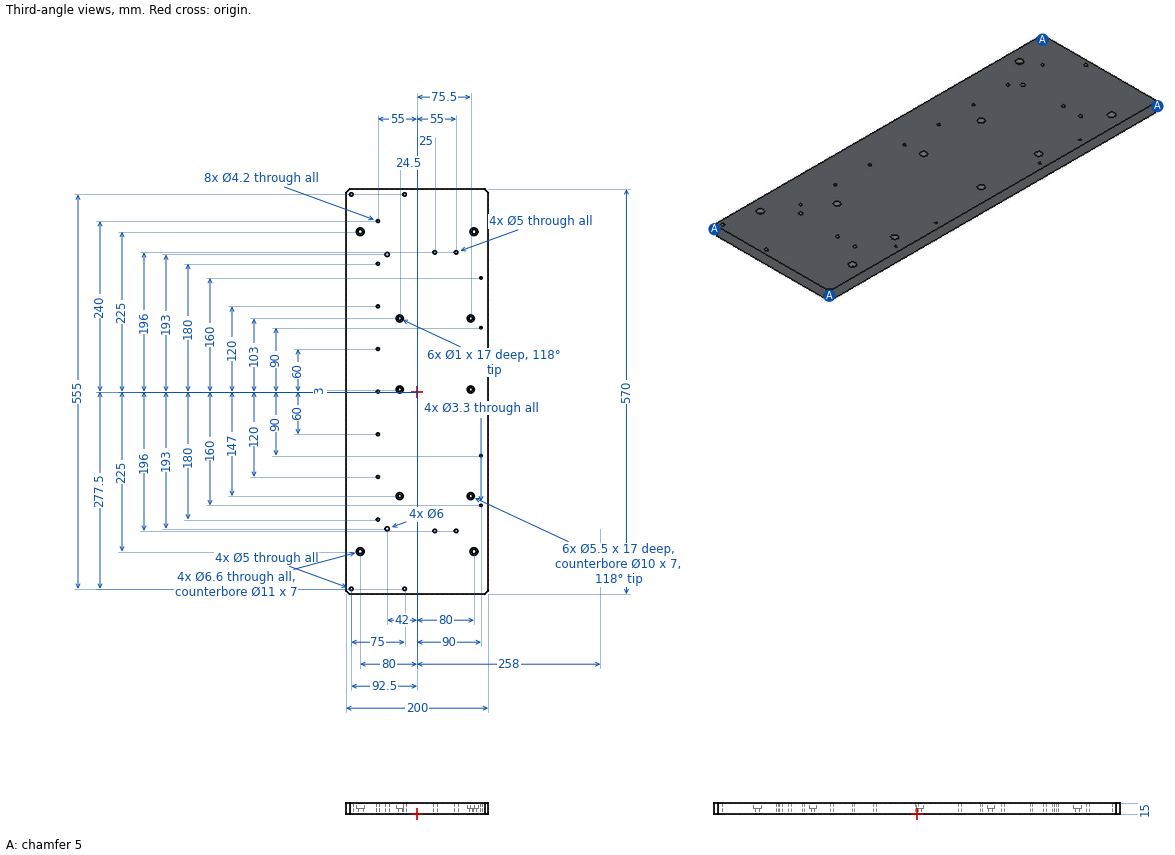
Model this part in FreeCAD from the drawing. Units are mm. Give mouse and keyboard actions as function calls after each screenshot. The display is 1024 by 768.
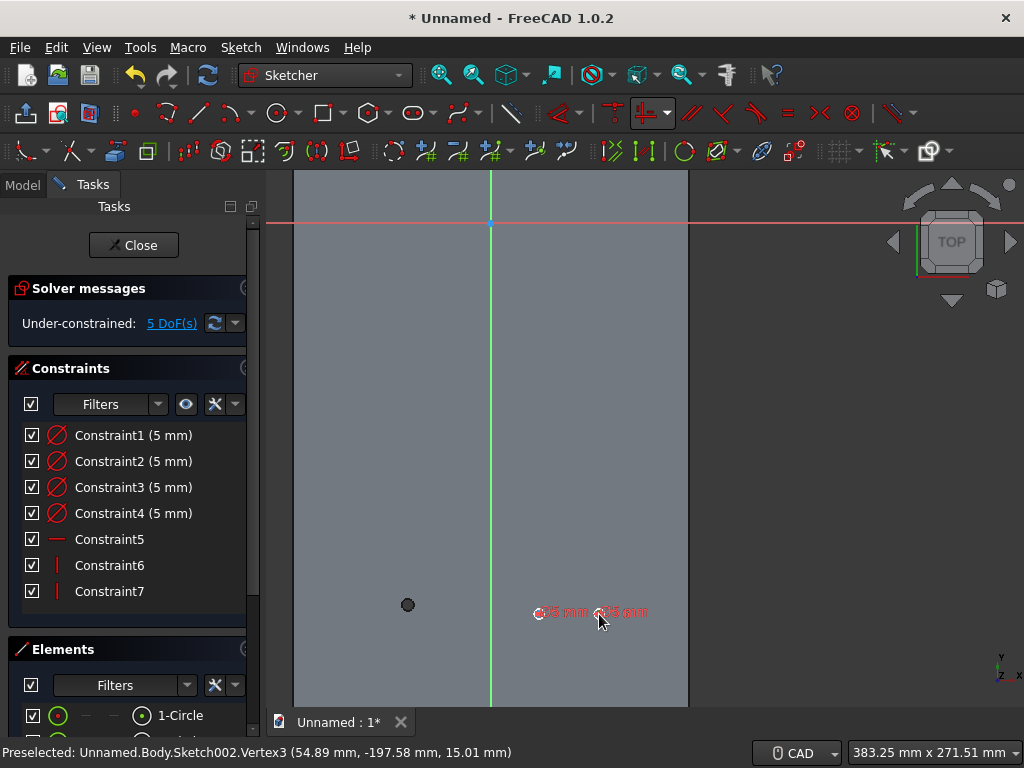
click(539, 614)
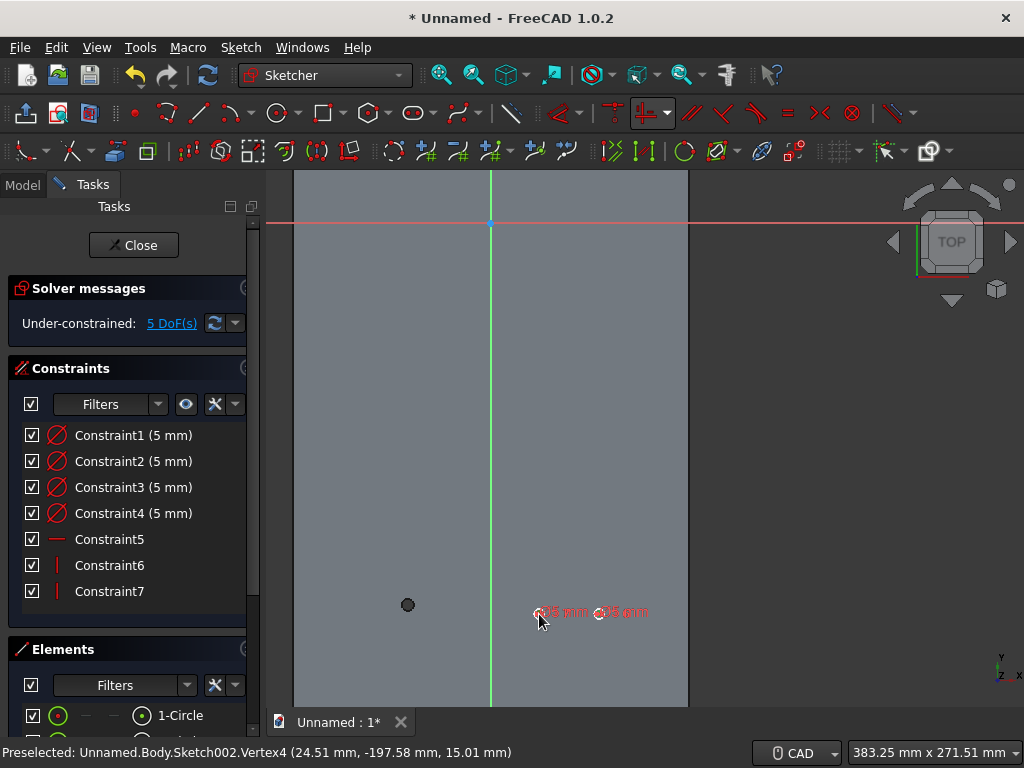
key(h)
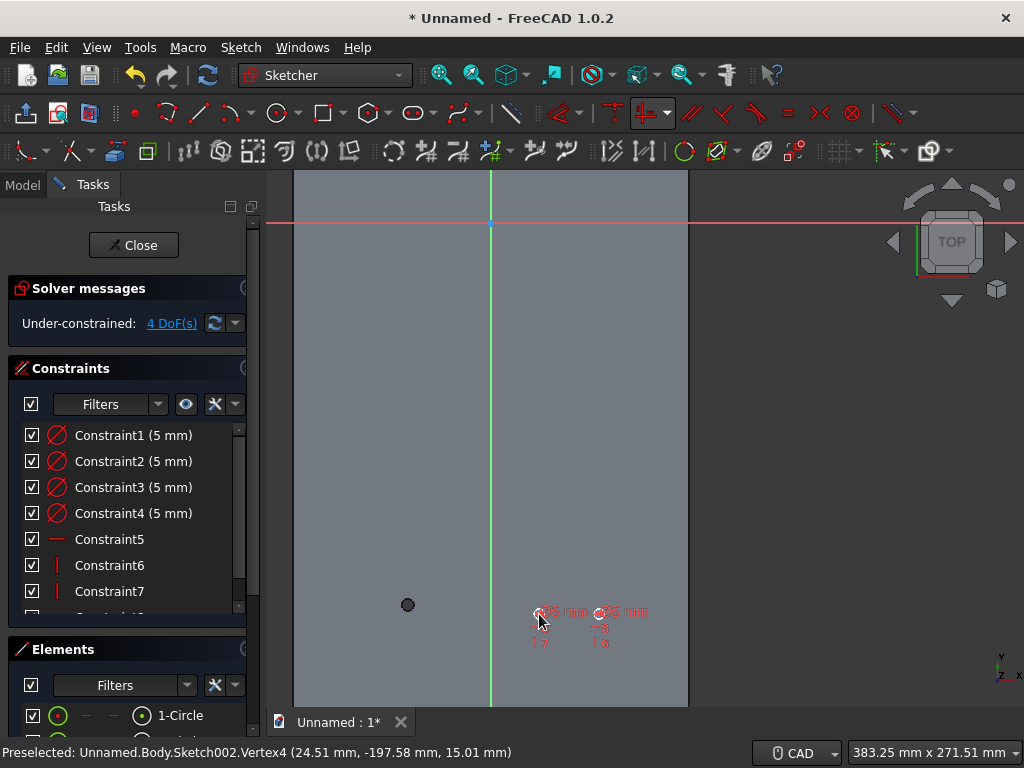
click(558, 114)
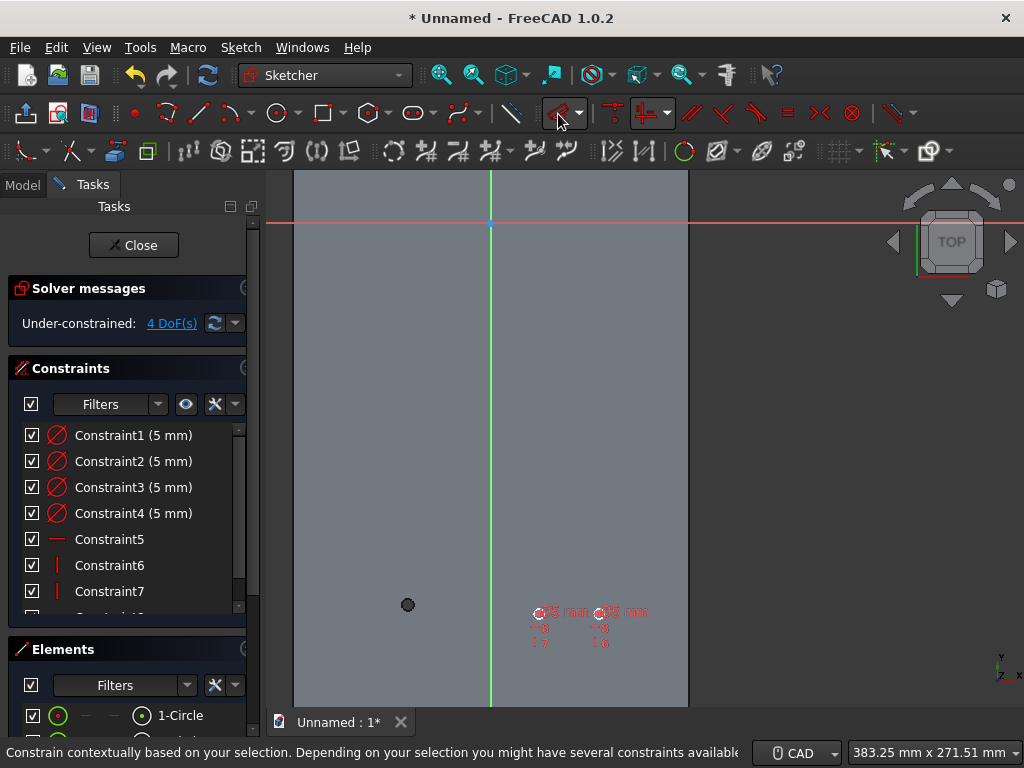
scroll(600, 614, down, 4)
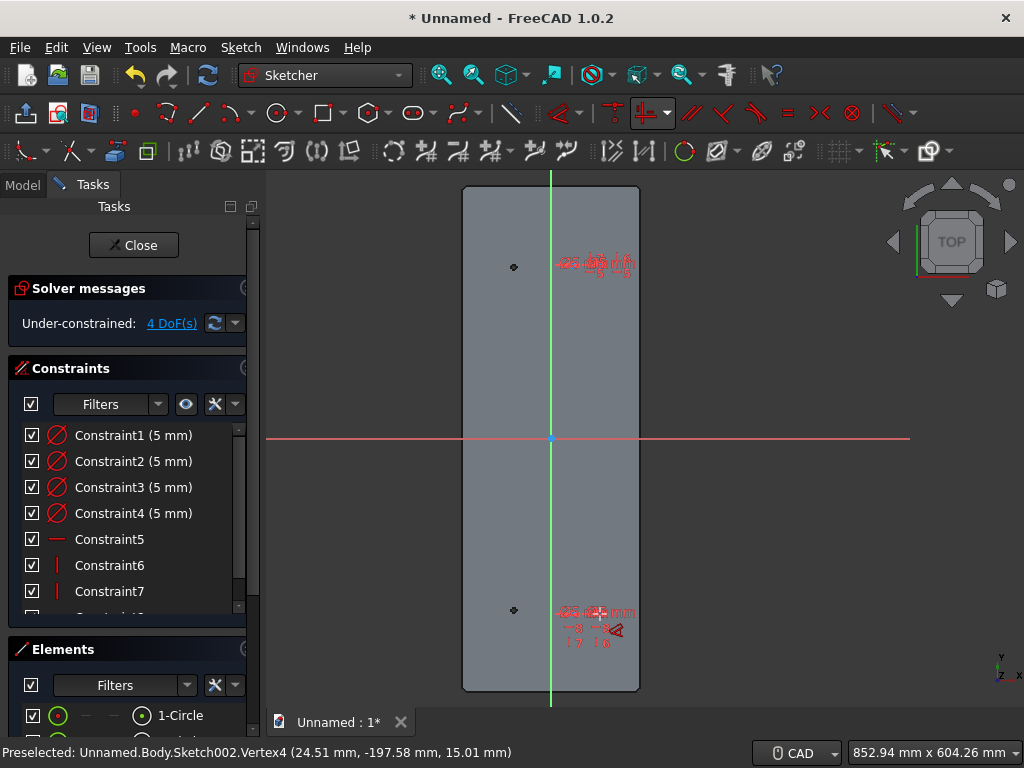
click(600, 265)
click(576, 231)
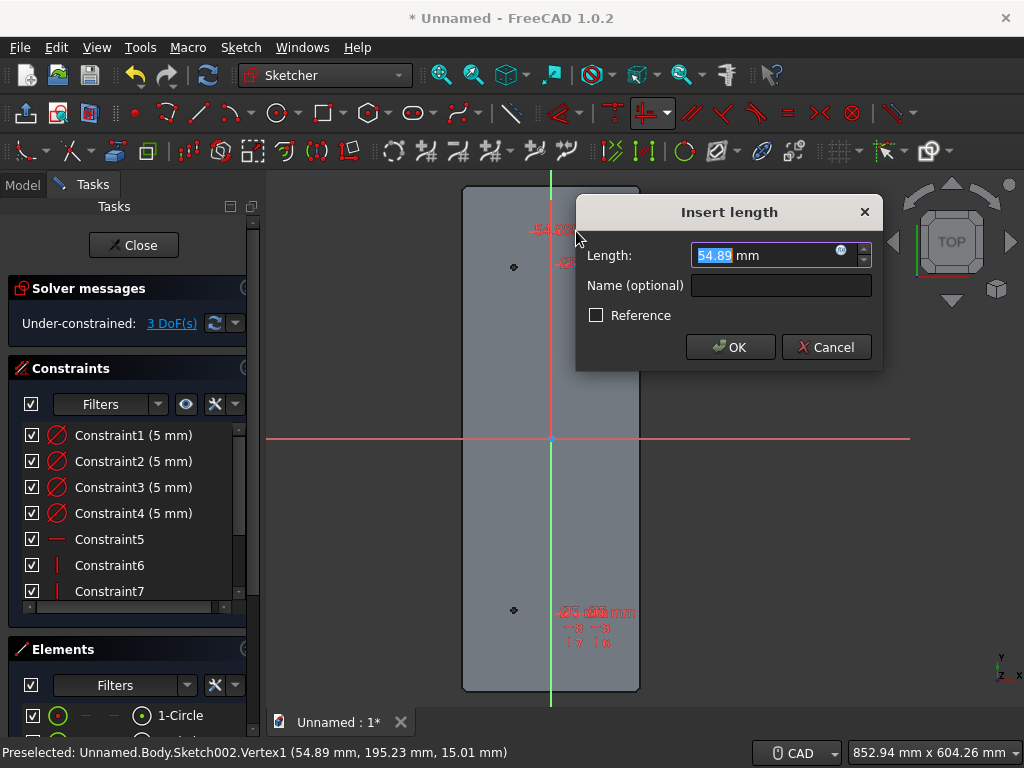
text(55)
key(Return)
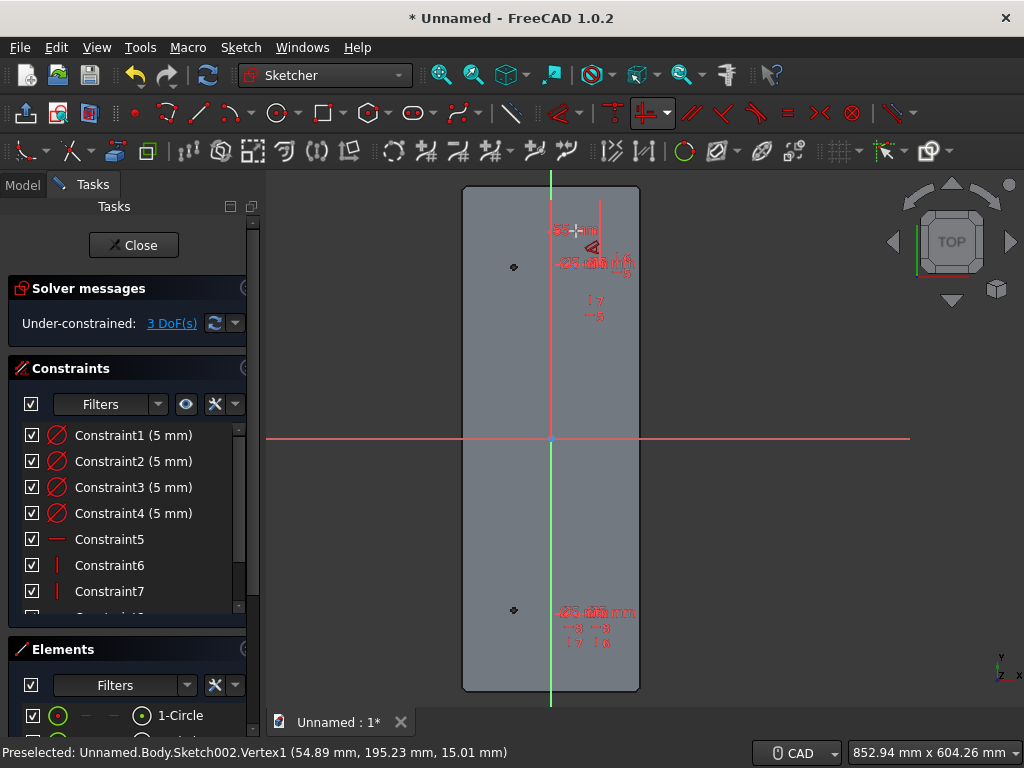
scroll(573, 265, up, 3)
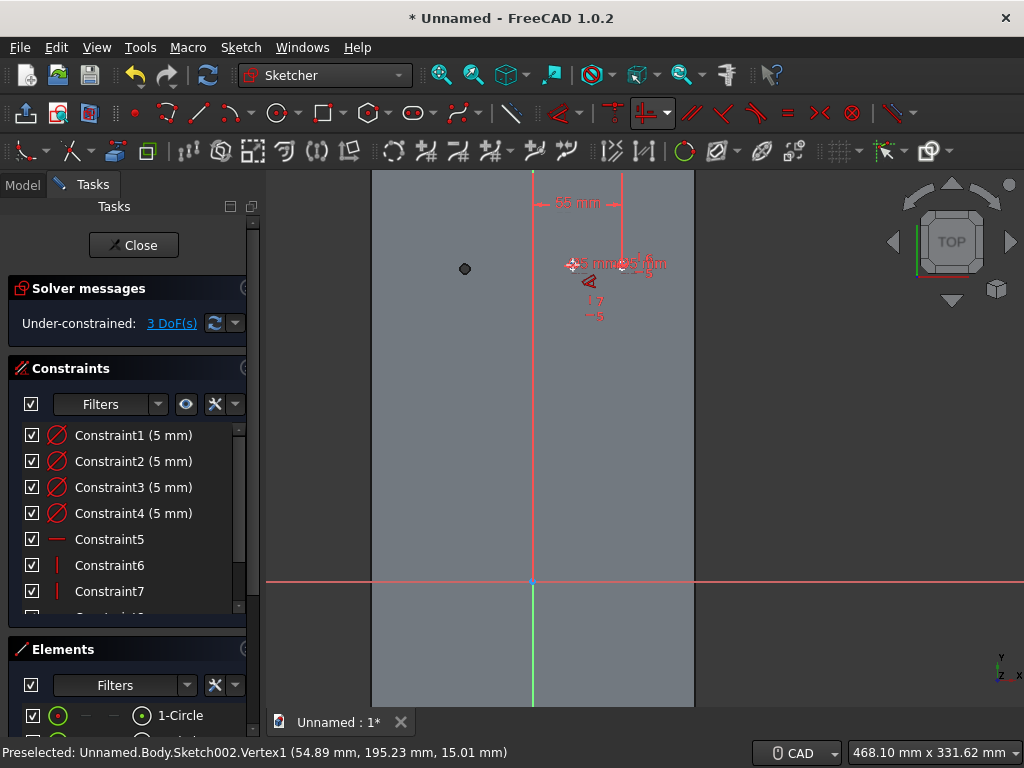
click(573, 266)
click(553, 232)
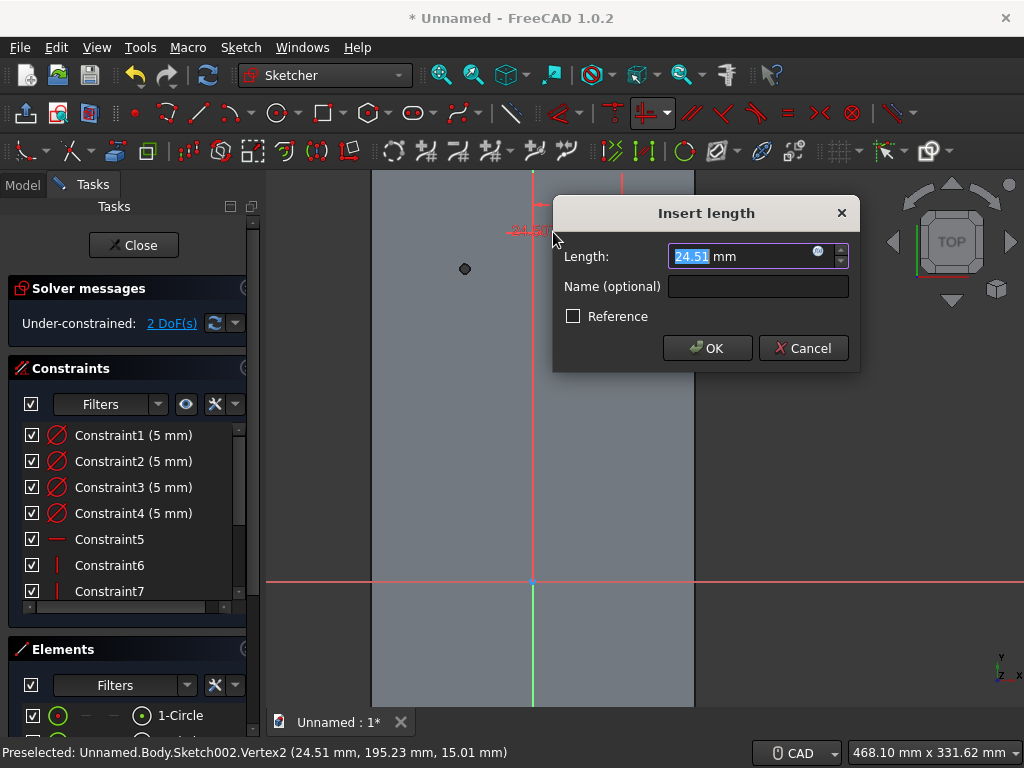
text(25)
key(Return)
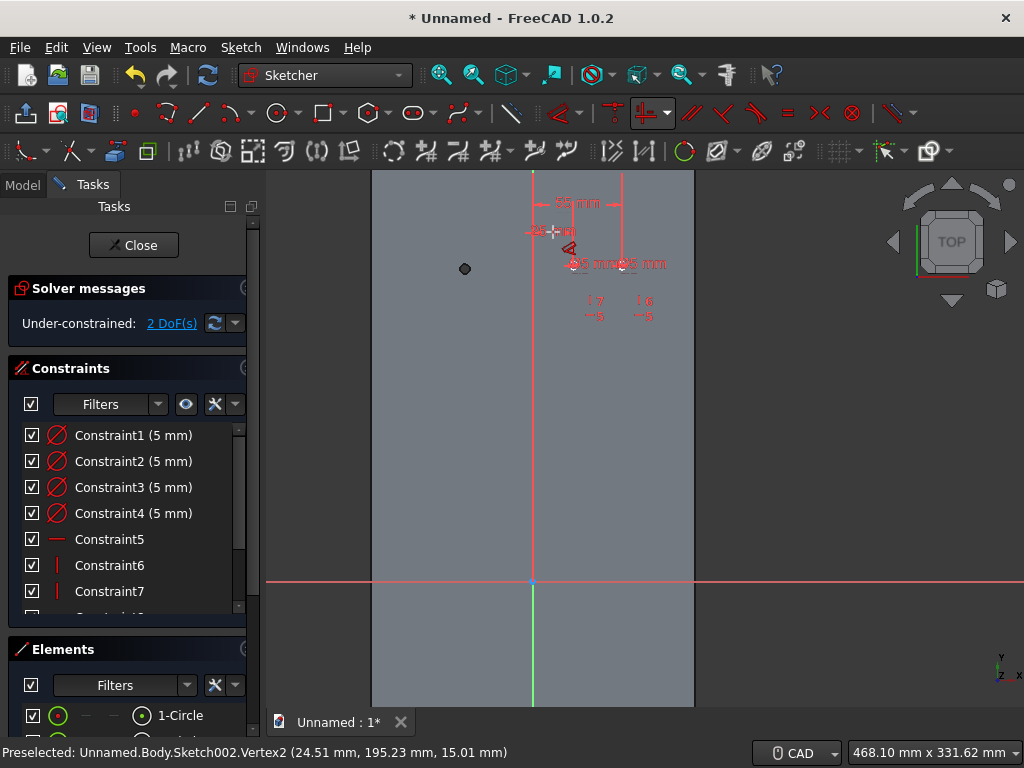
click(622, 266)
click(499, 424)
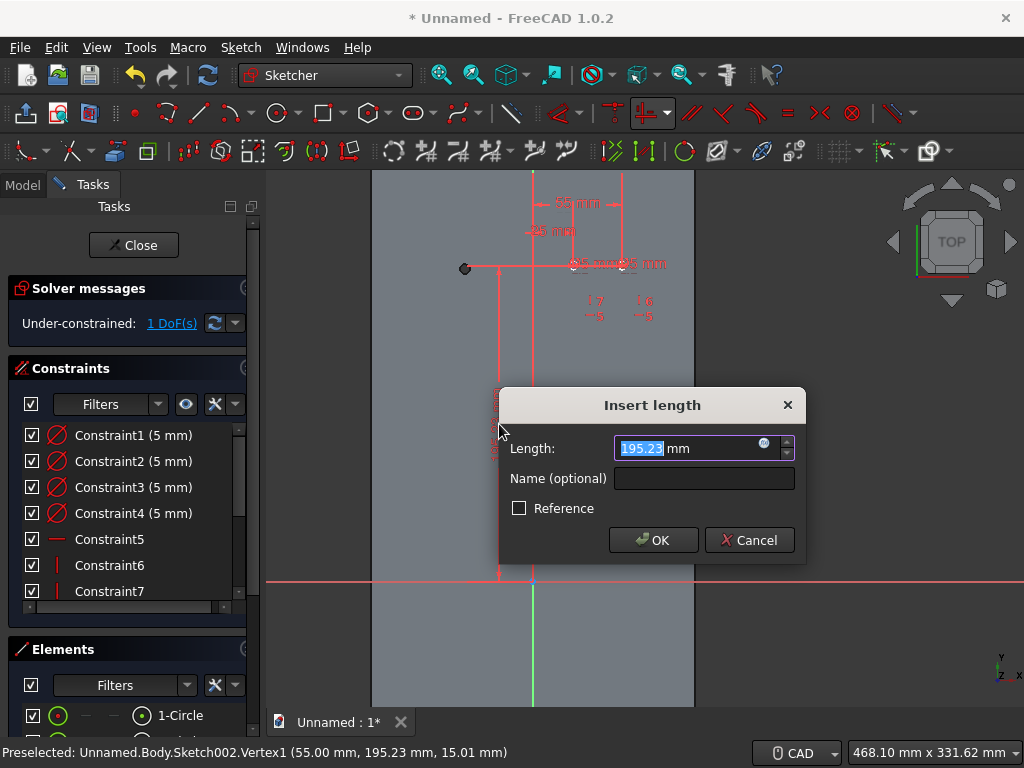
text(196)
key(Return)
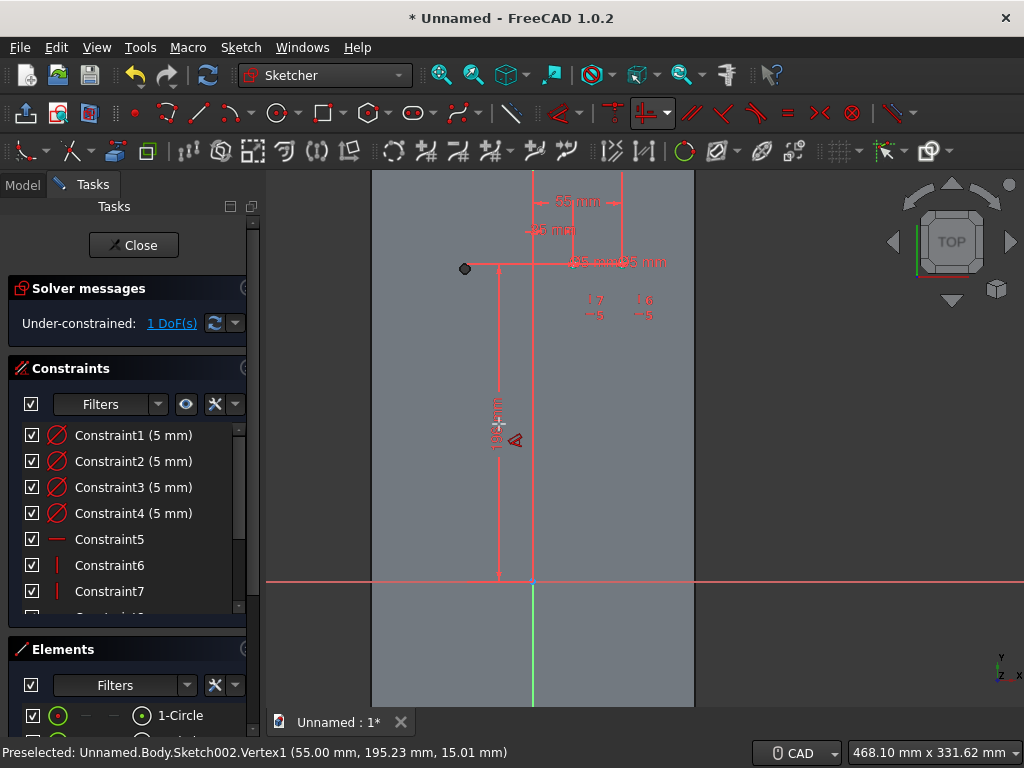
scroll(573, 264, down, 3)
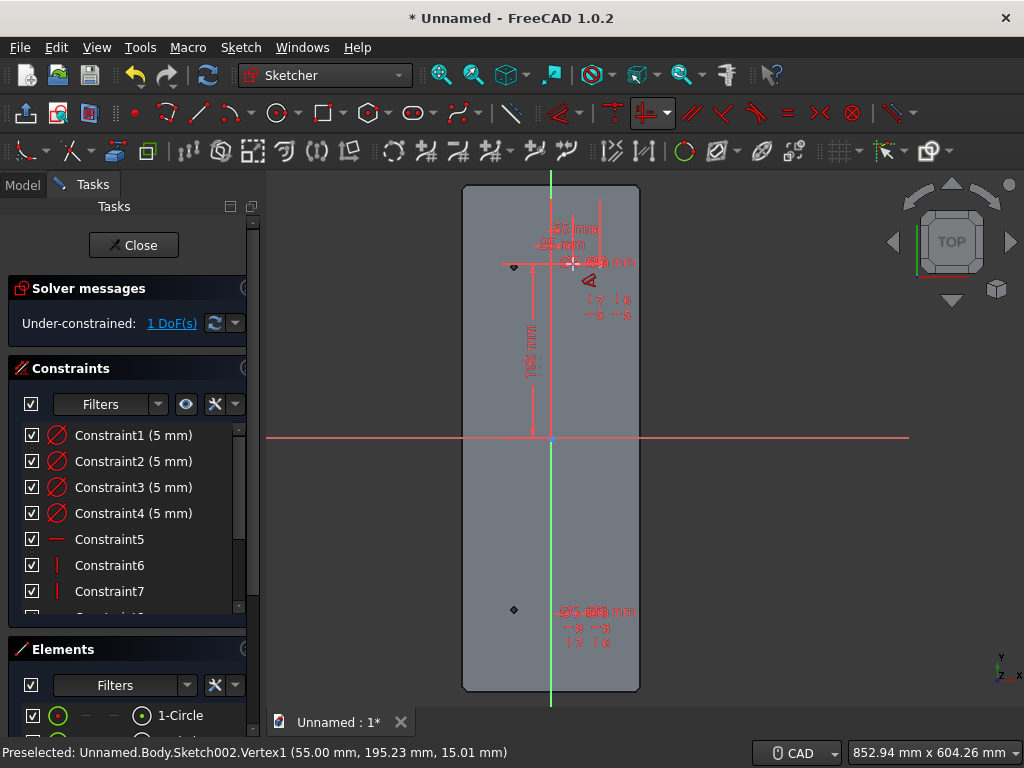
click(600, 614)
click(517, 526)